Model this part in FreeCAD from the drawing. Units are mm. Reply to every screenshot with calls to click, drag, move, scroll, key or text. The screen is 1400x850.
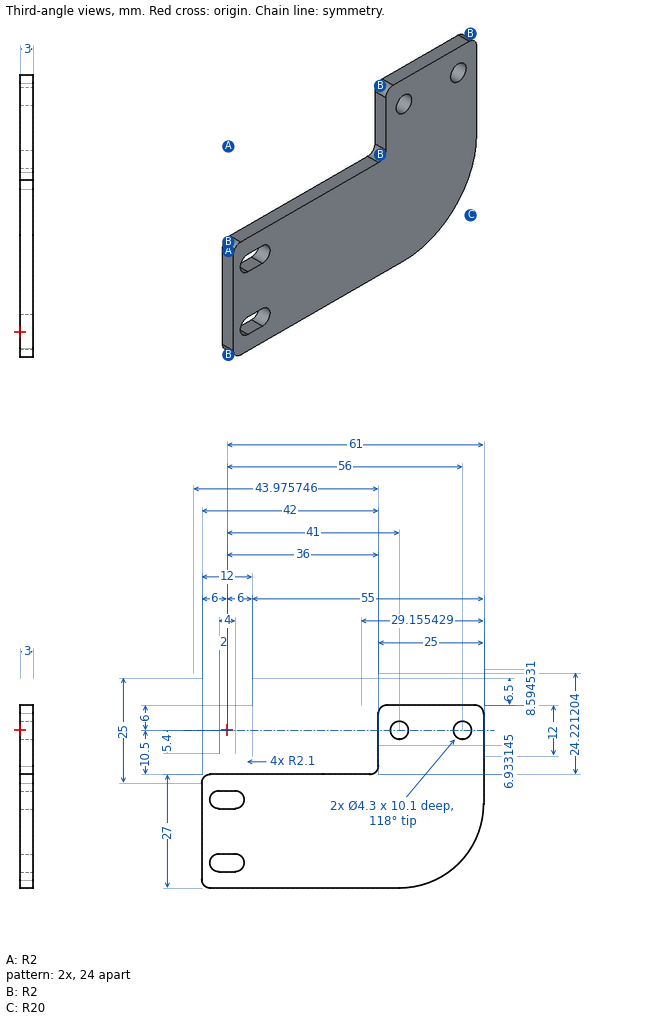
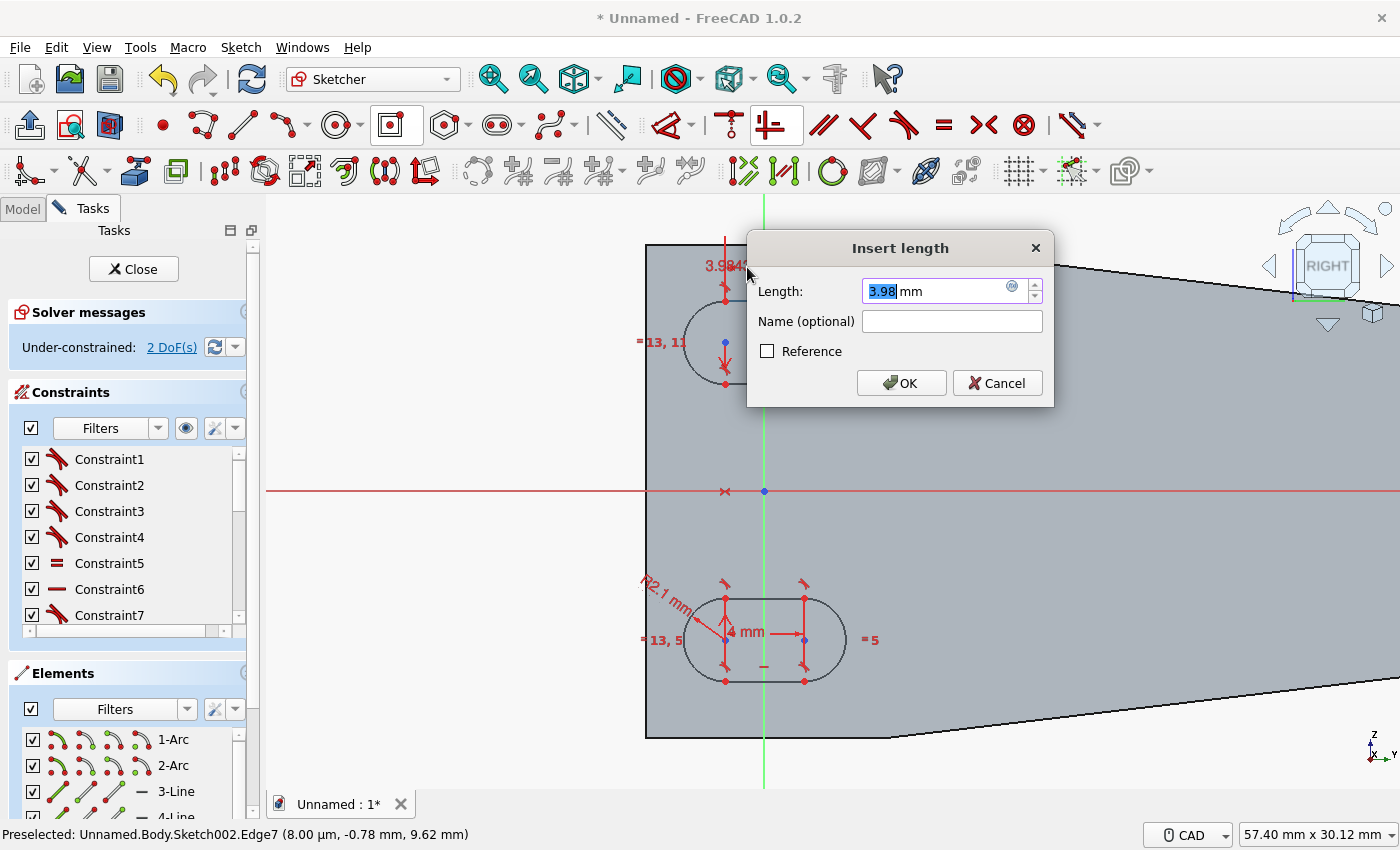
text(4)
key(Return)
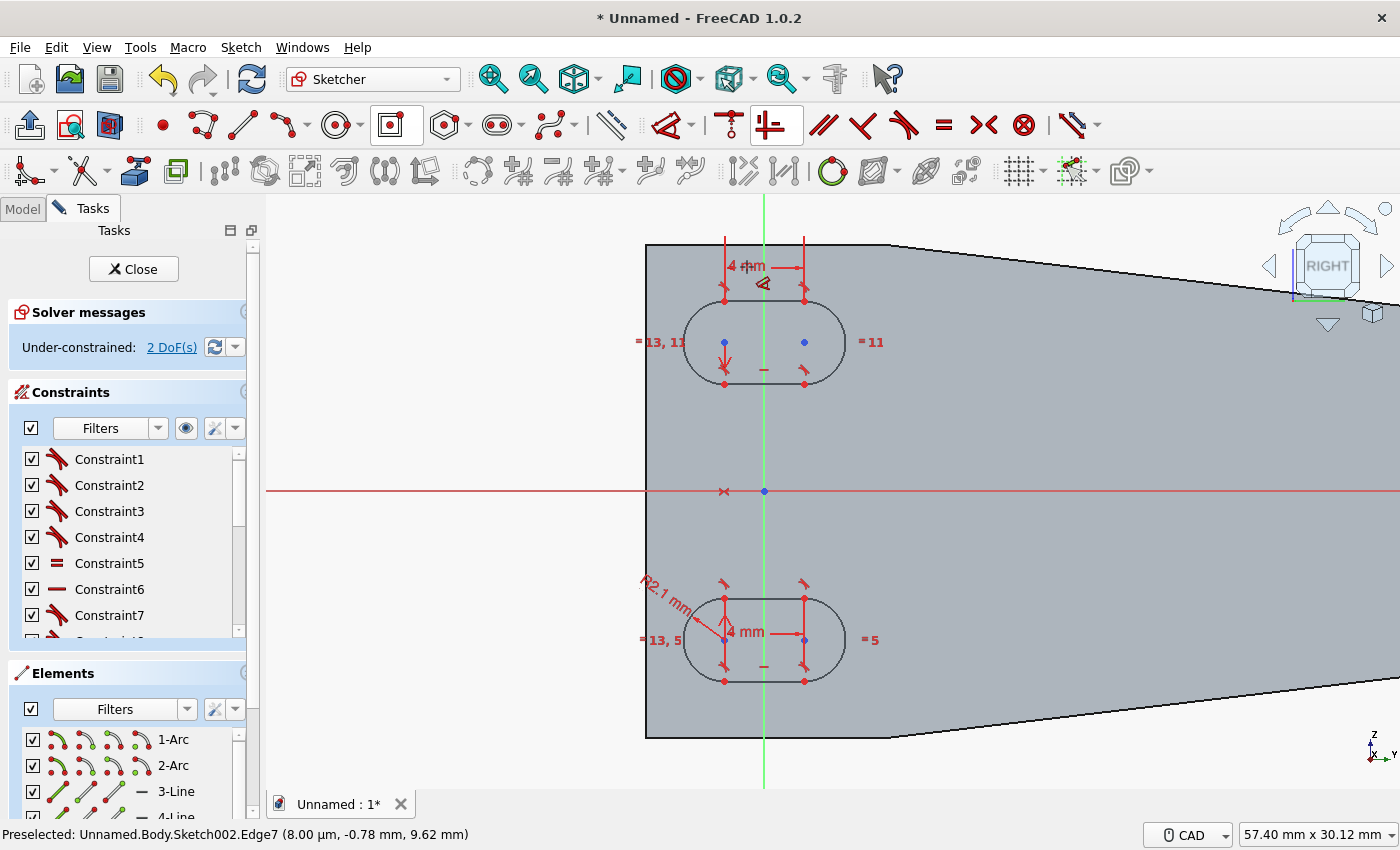
click(725, 599)
click(745, 457)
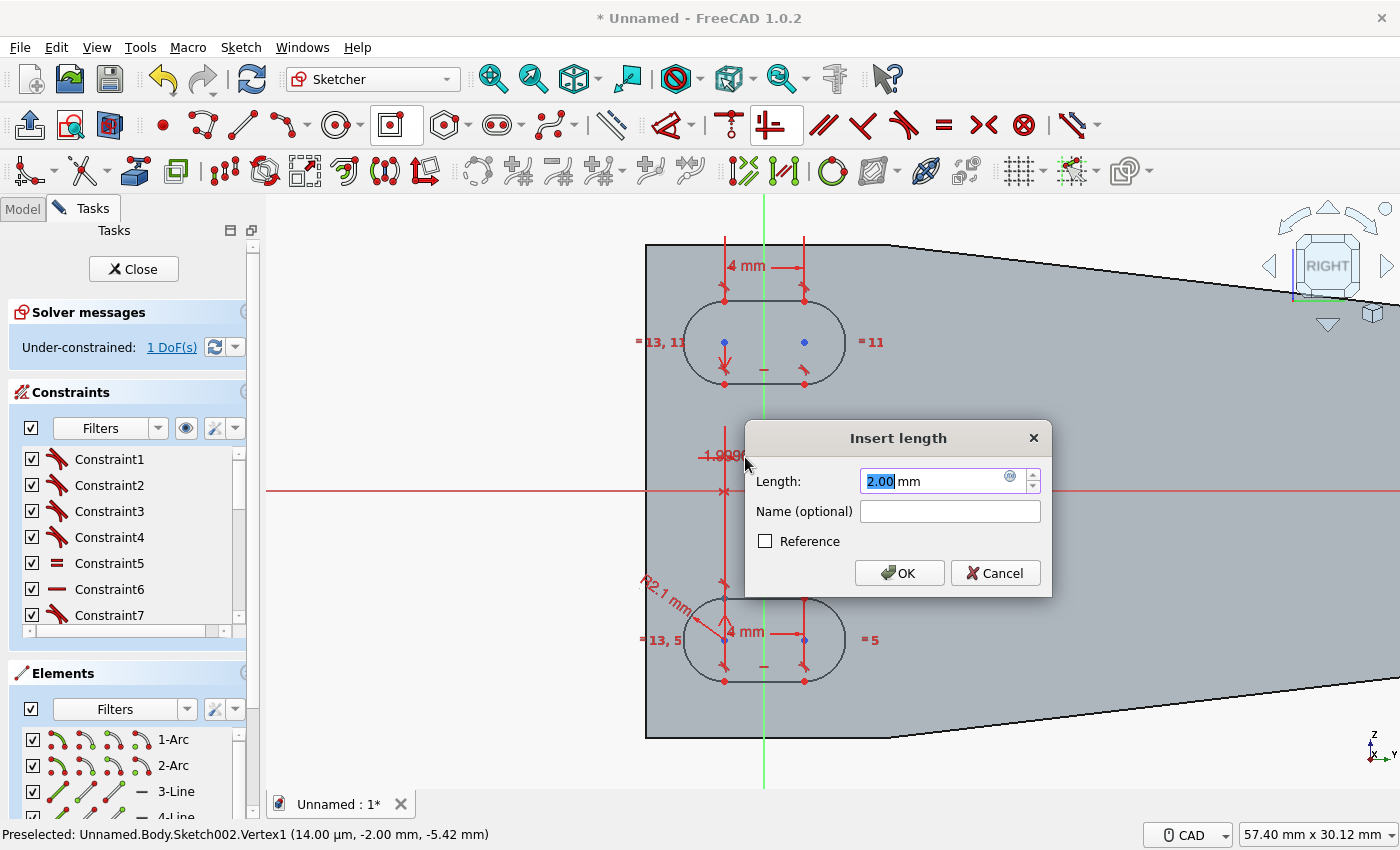
text(2)
key(Return)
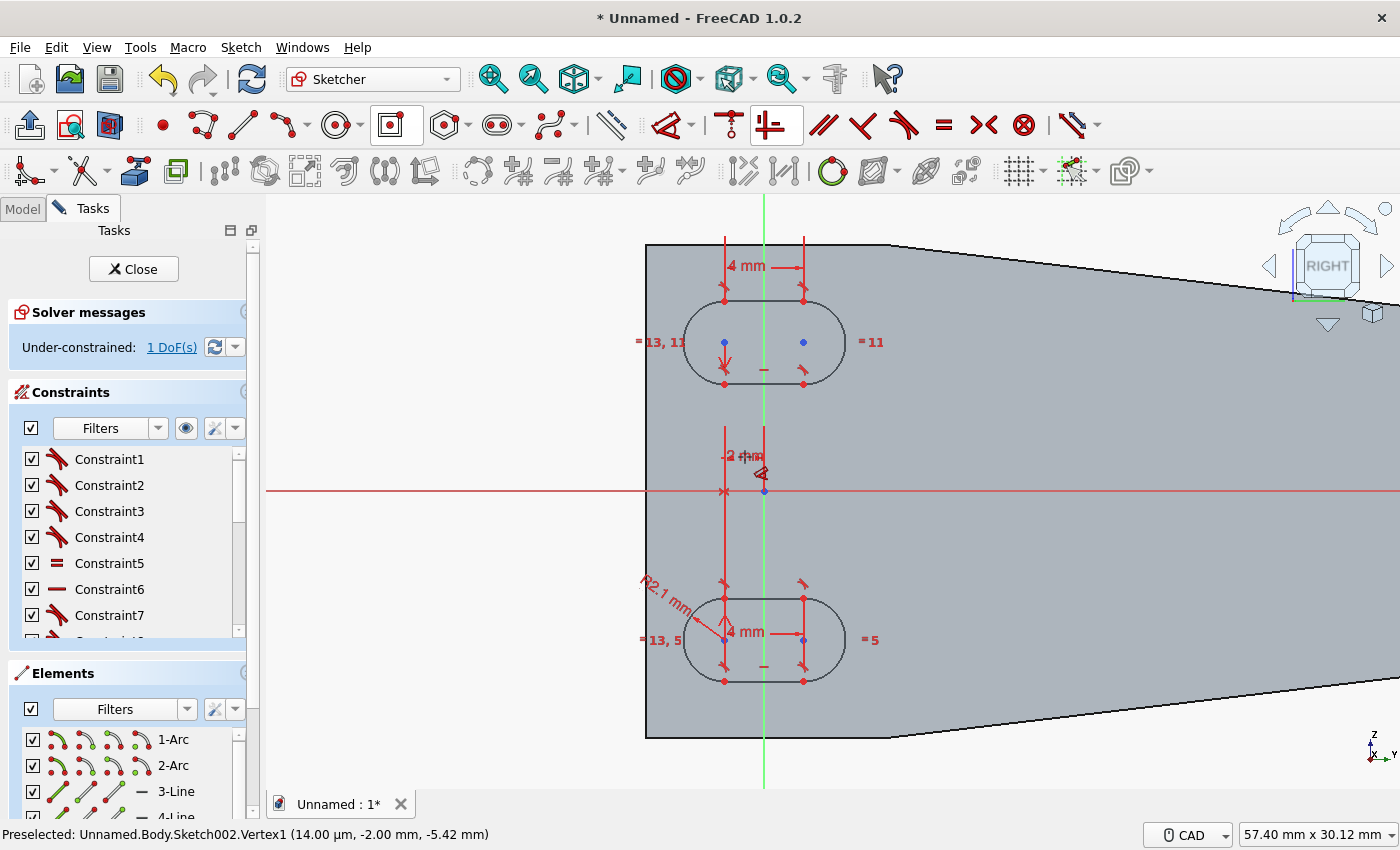
click(725, 599)
click(691, 545)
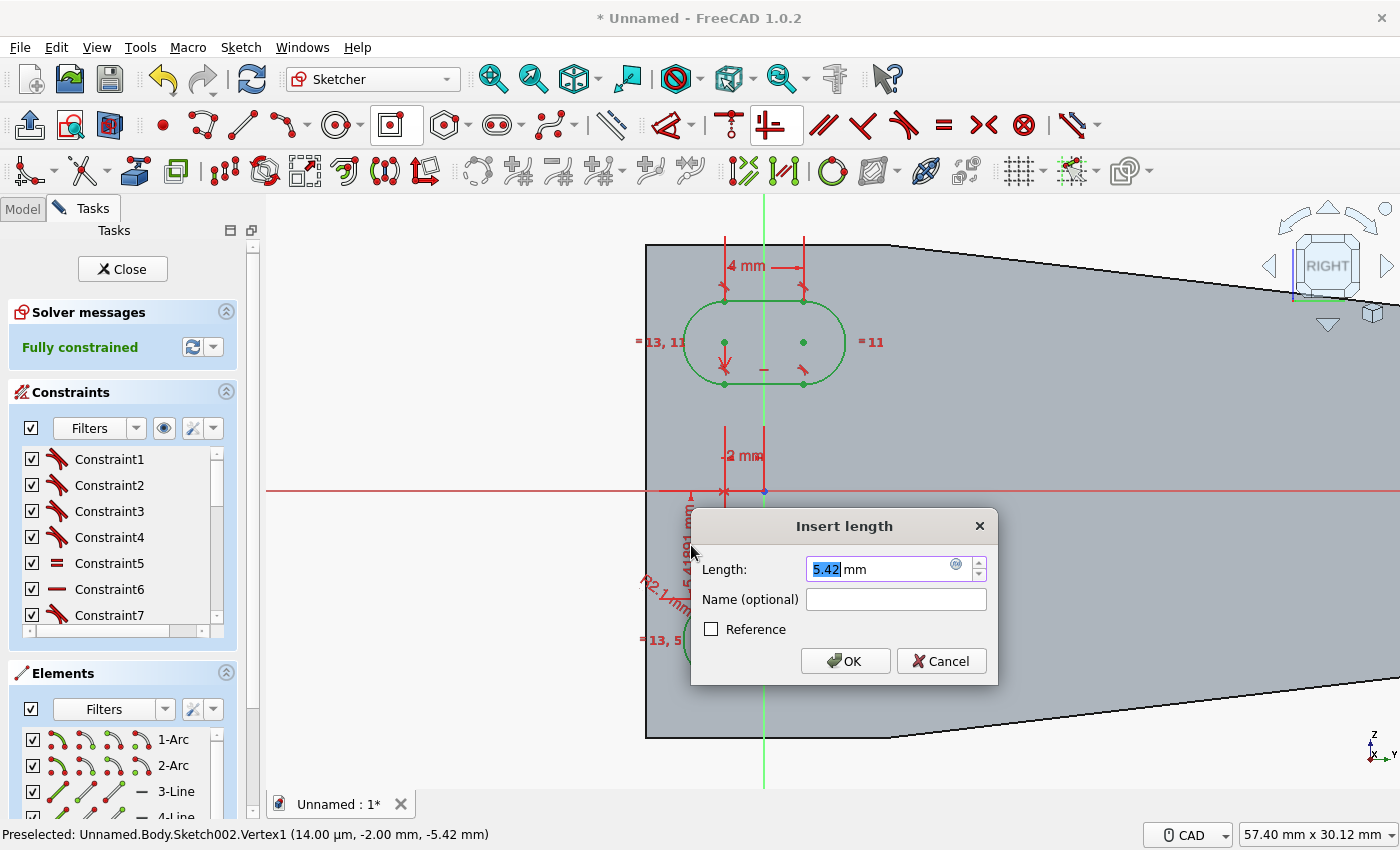
text(5.4)
key(Return)
key(Escape)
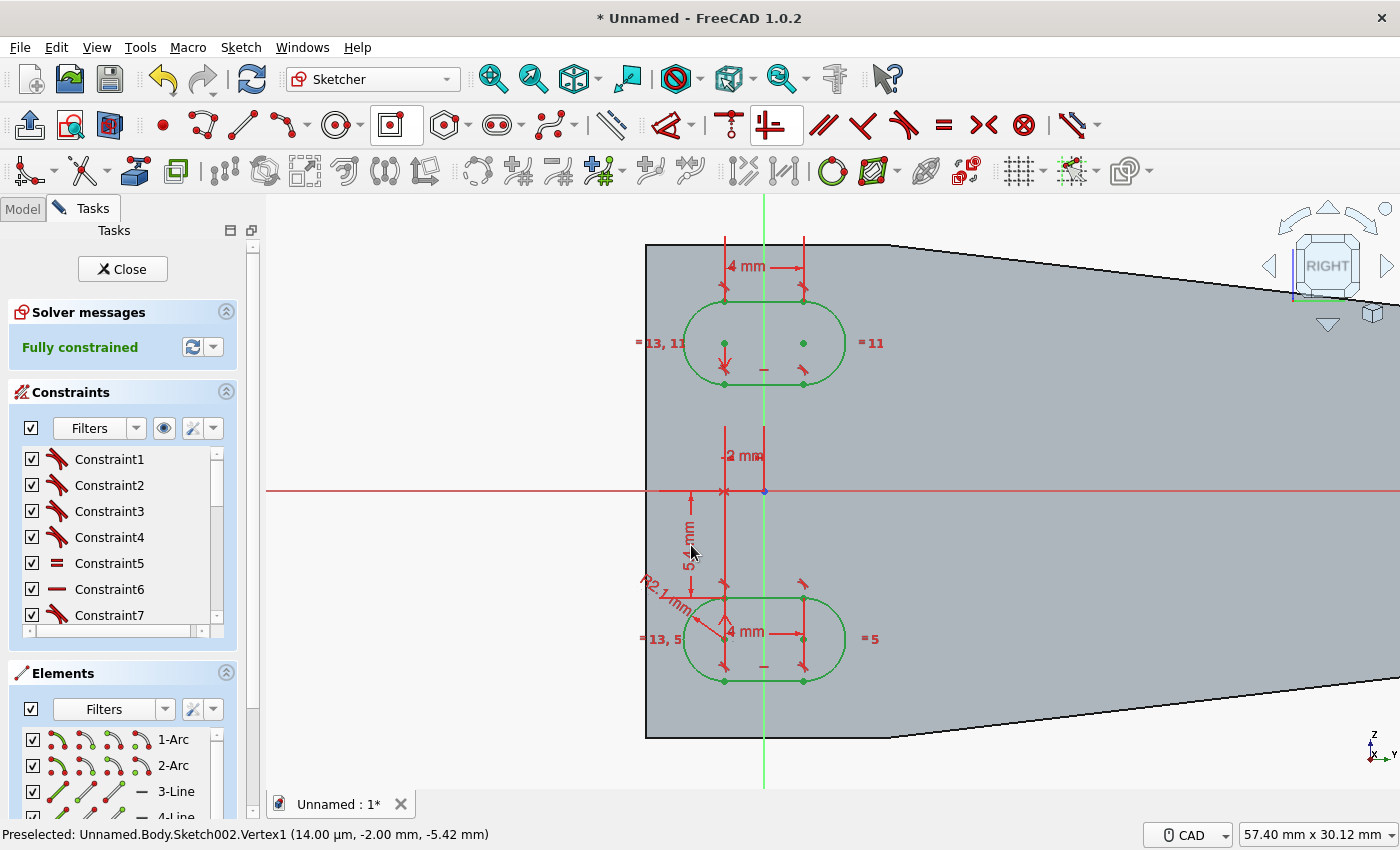
click(123, 269)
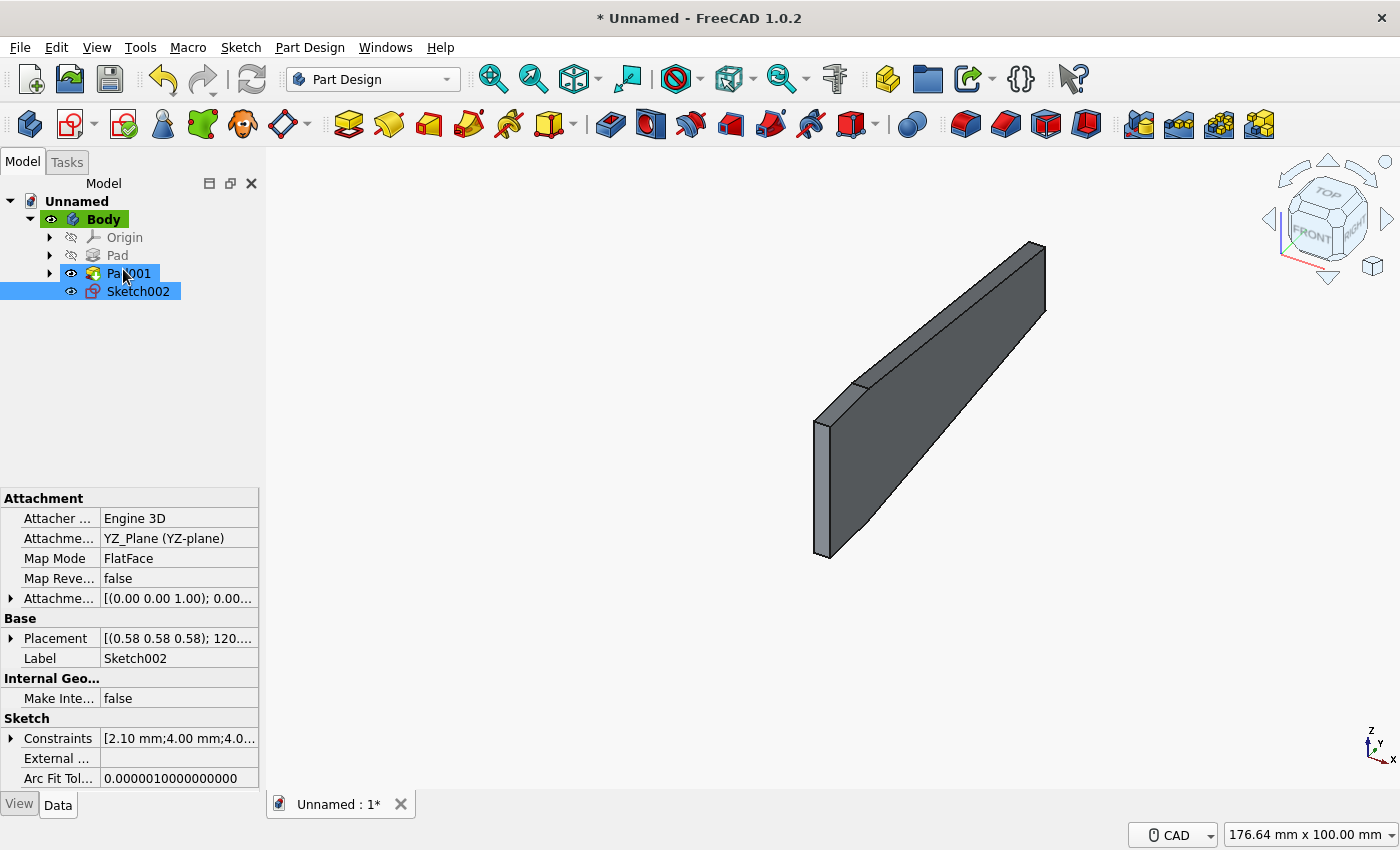
click(612, 124)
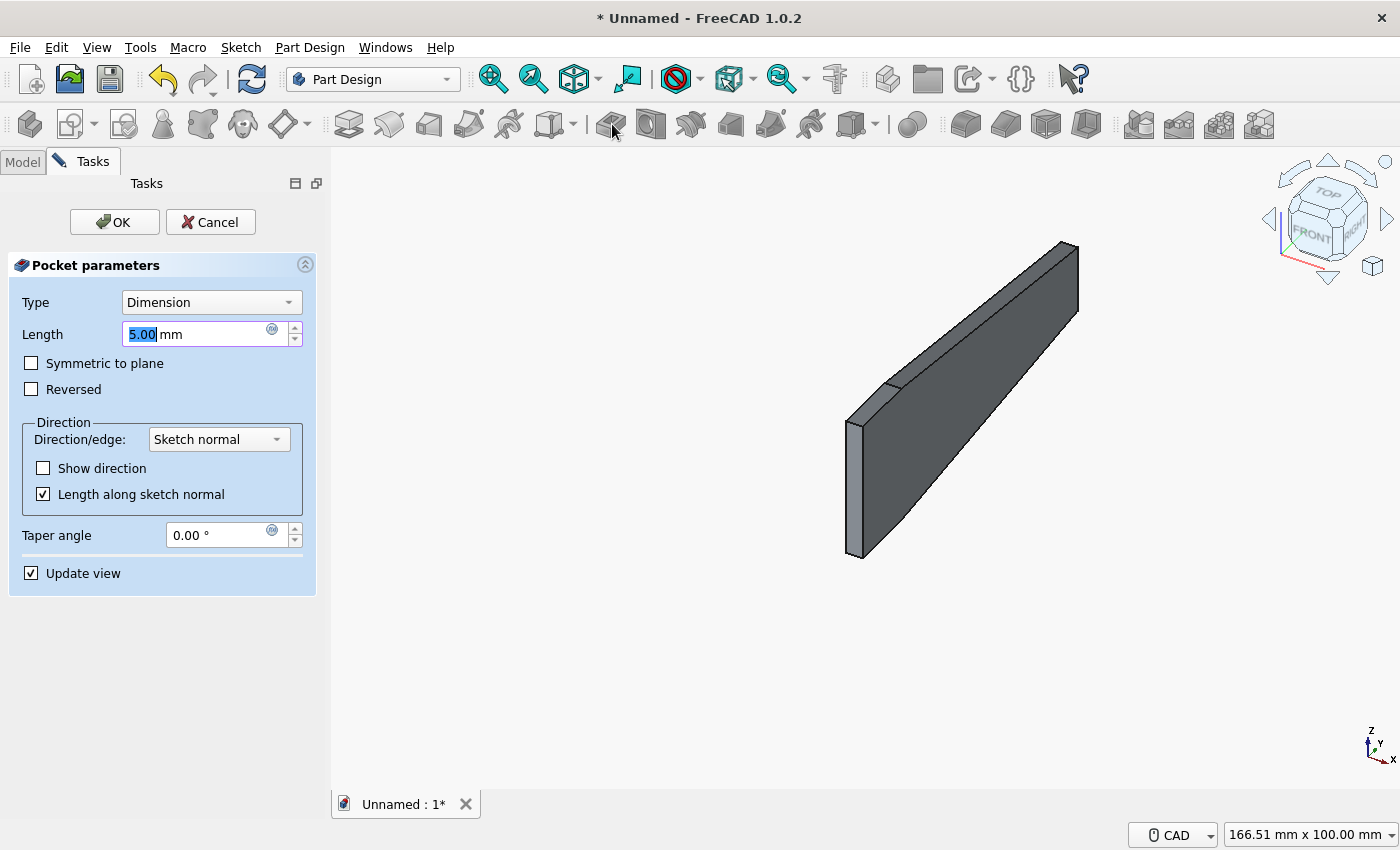
text(3)
key(Tab)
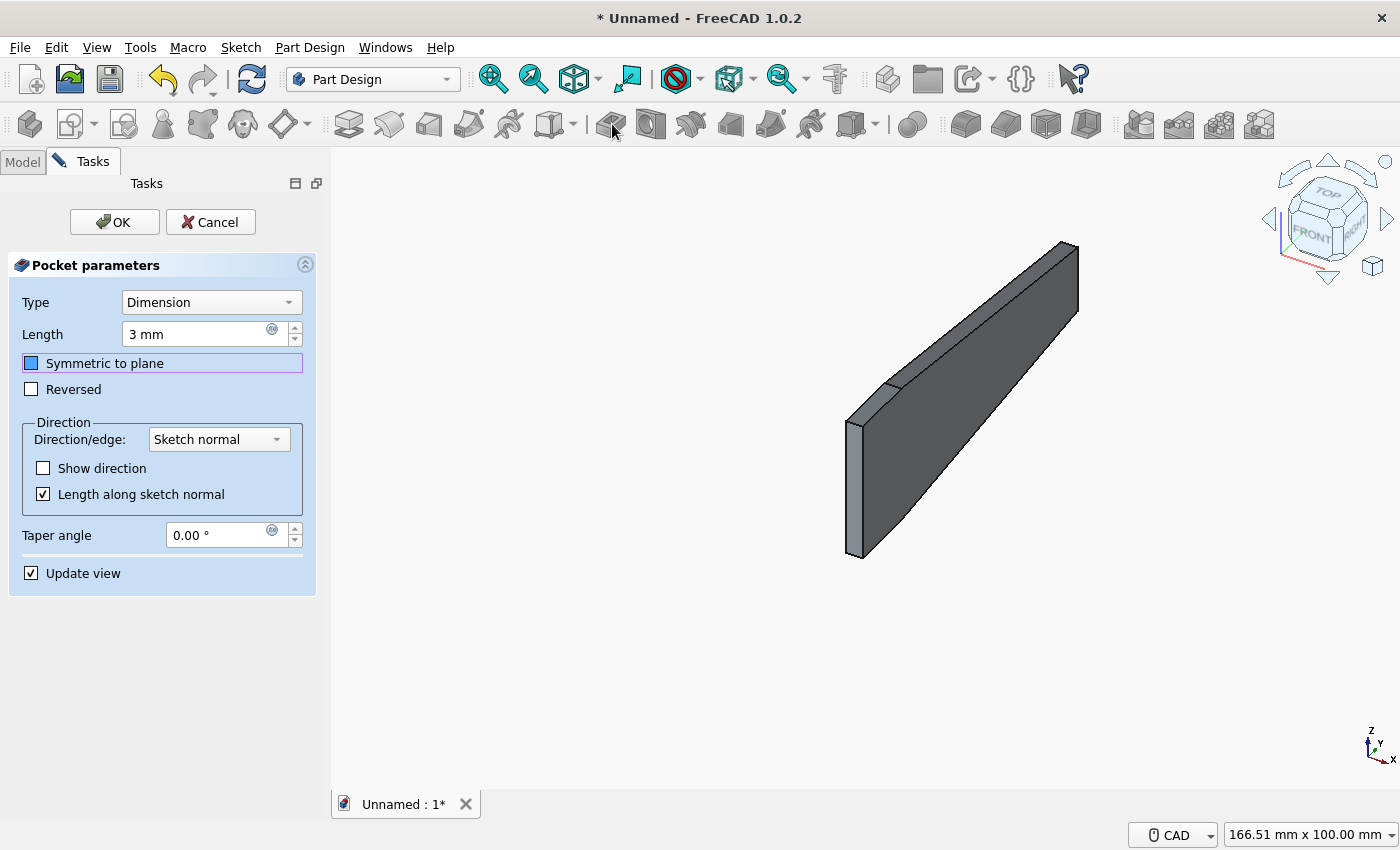
click(30, 389)